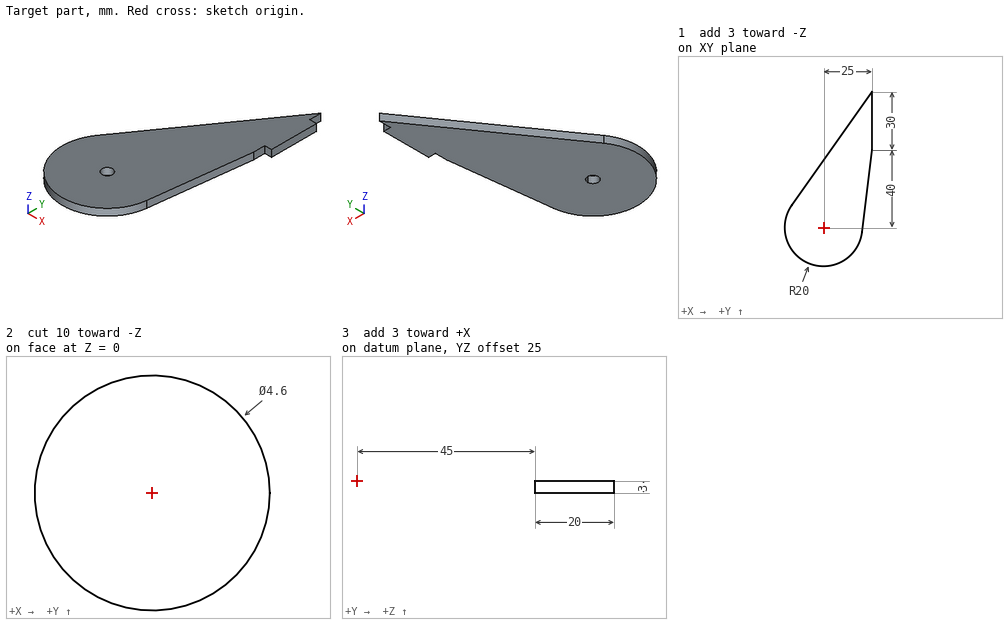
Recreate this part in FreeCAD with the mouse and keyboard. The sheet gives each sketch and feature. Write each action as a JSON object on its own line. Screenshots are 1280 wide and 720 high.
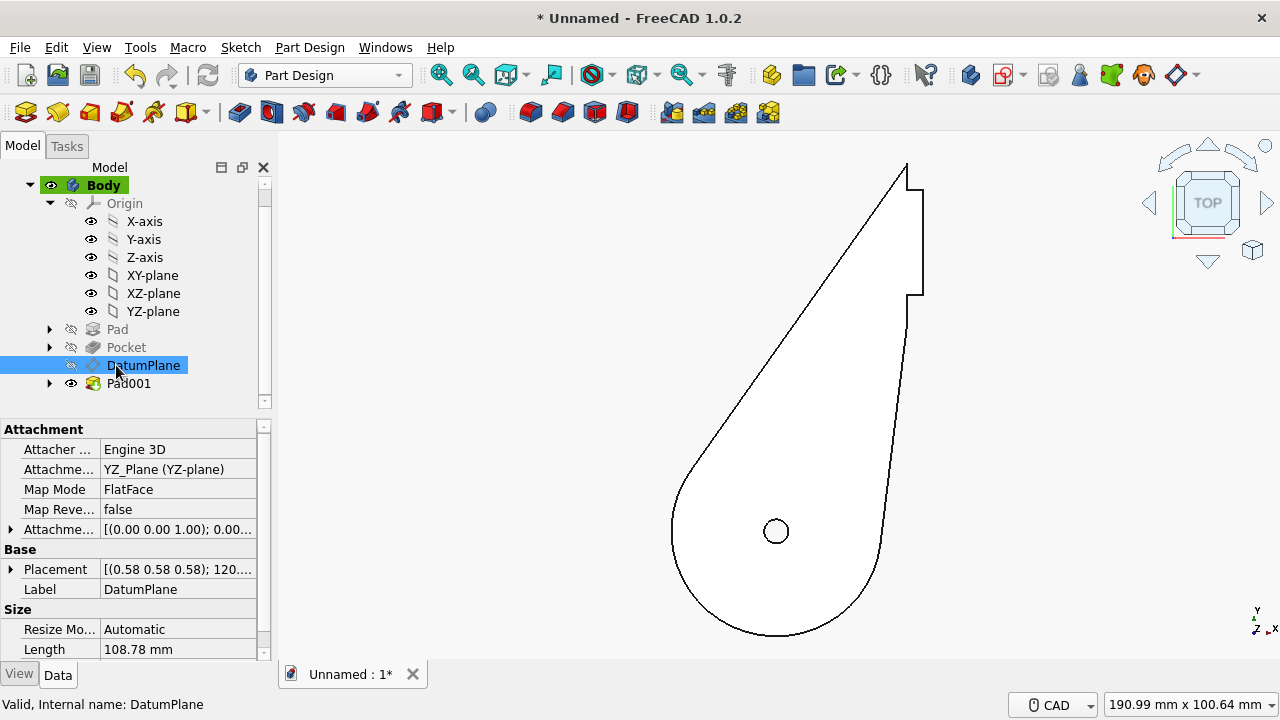
{"action": "key", "text": "0"}